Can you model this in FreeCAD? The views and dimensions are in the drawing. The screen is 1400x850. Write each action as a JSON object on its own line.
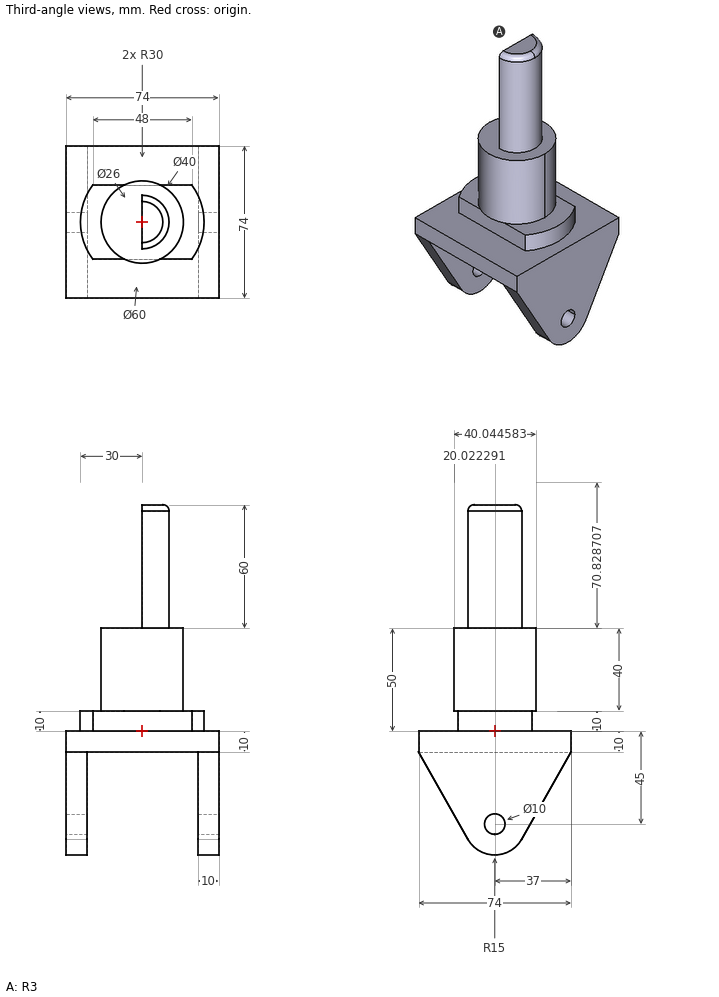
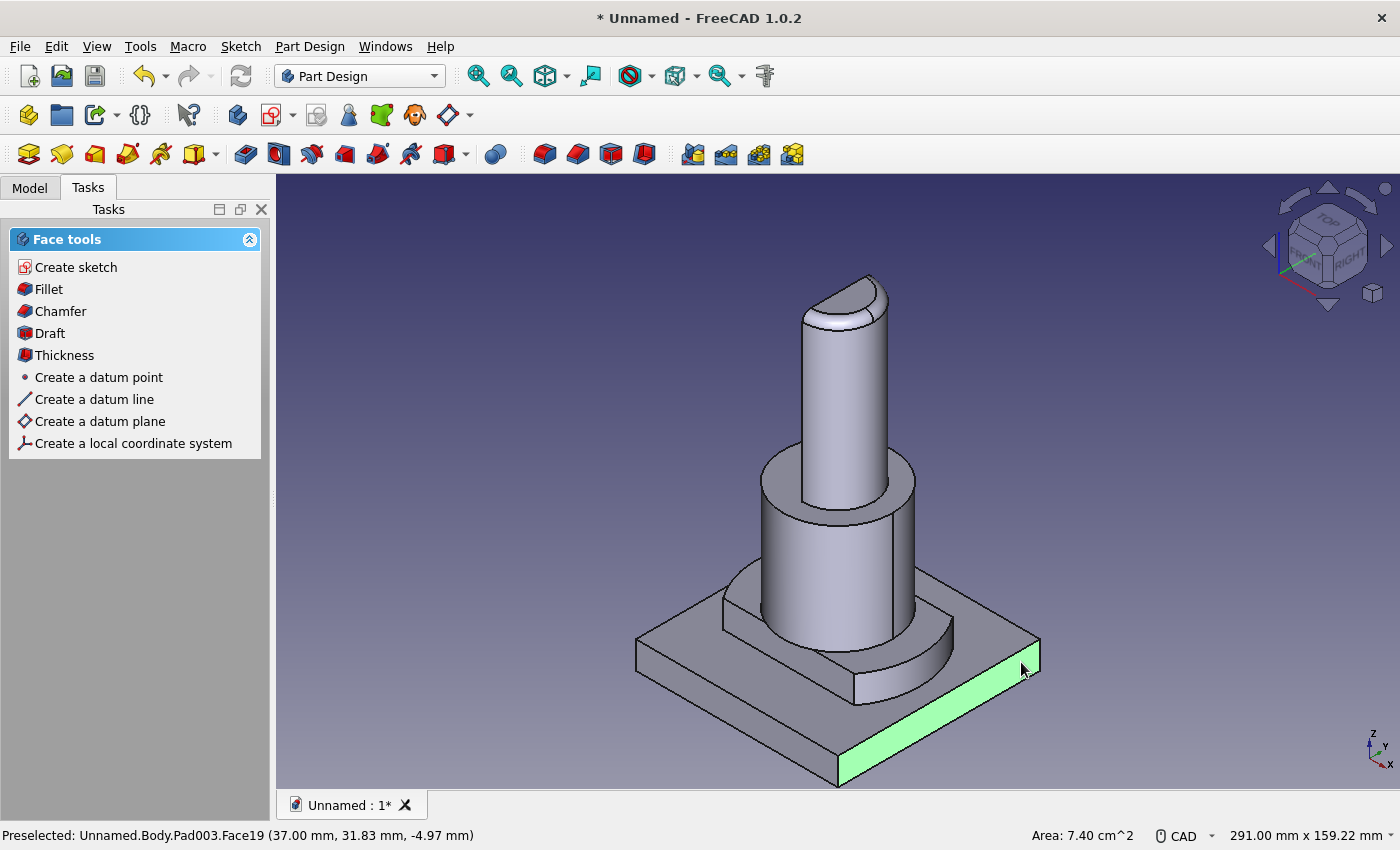
{"action": "left_click", "coordinate": [270, 116]}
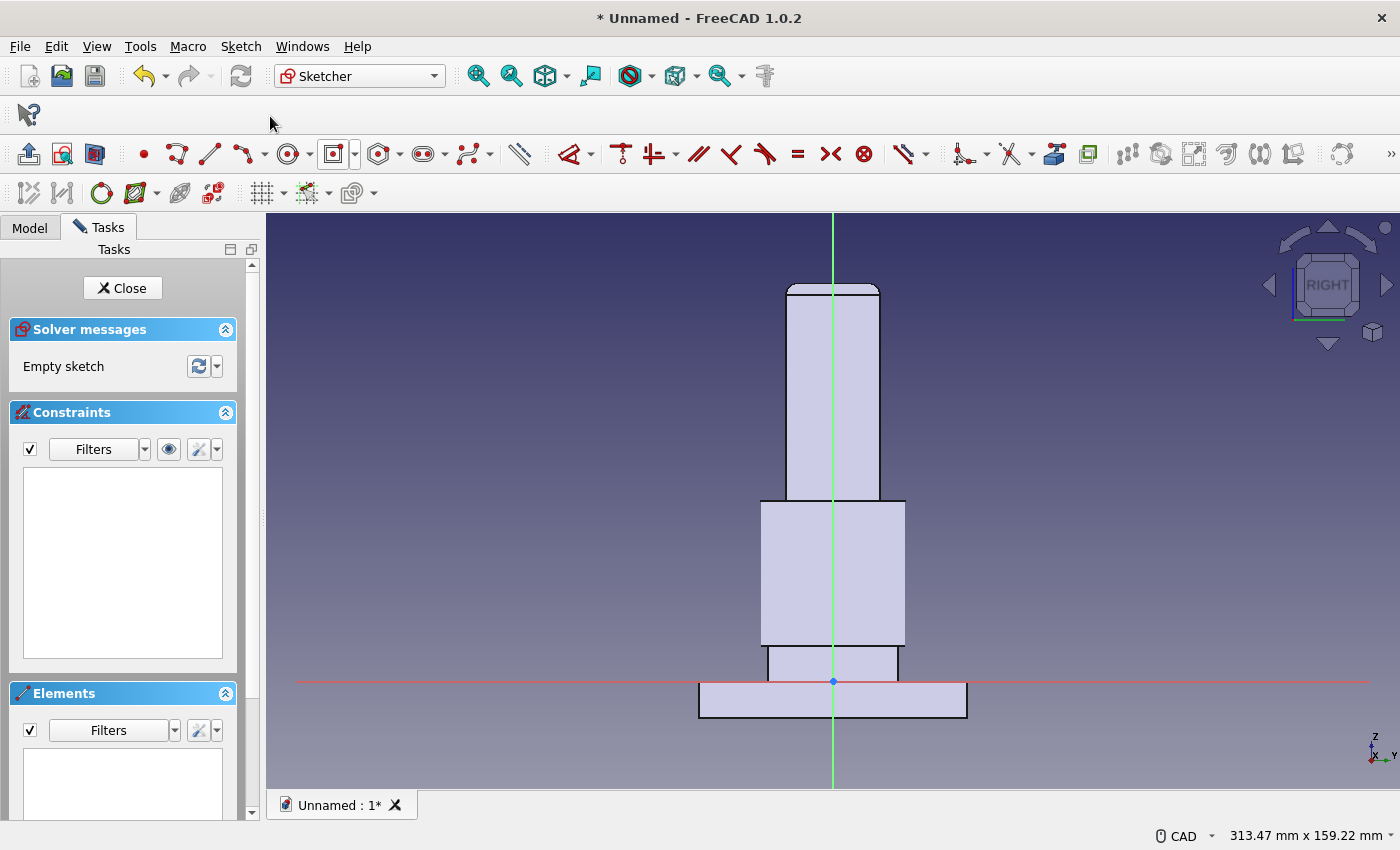
{"action": "scroll", "coordinate": [764, 501], "scroll_direction": "down", "scroll_amount": 5}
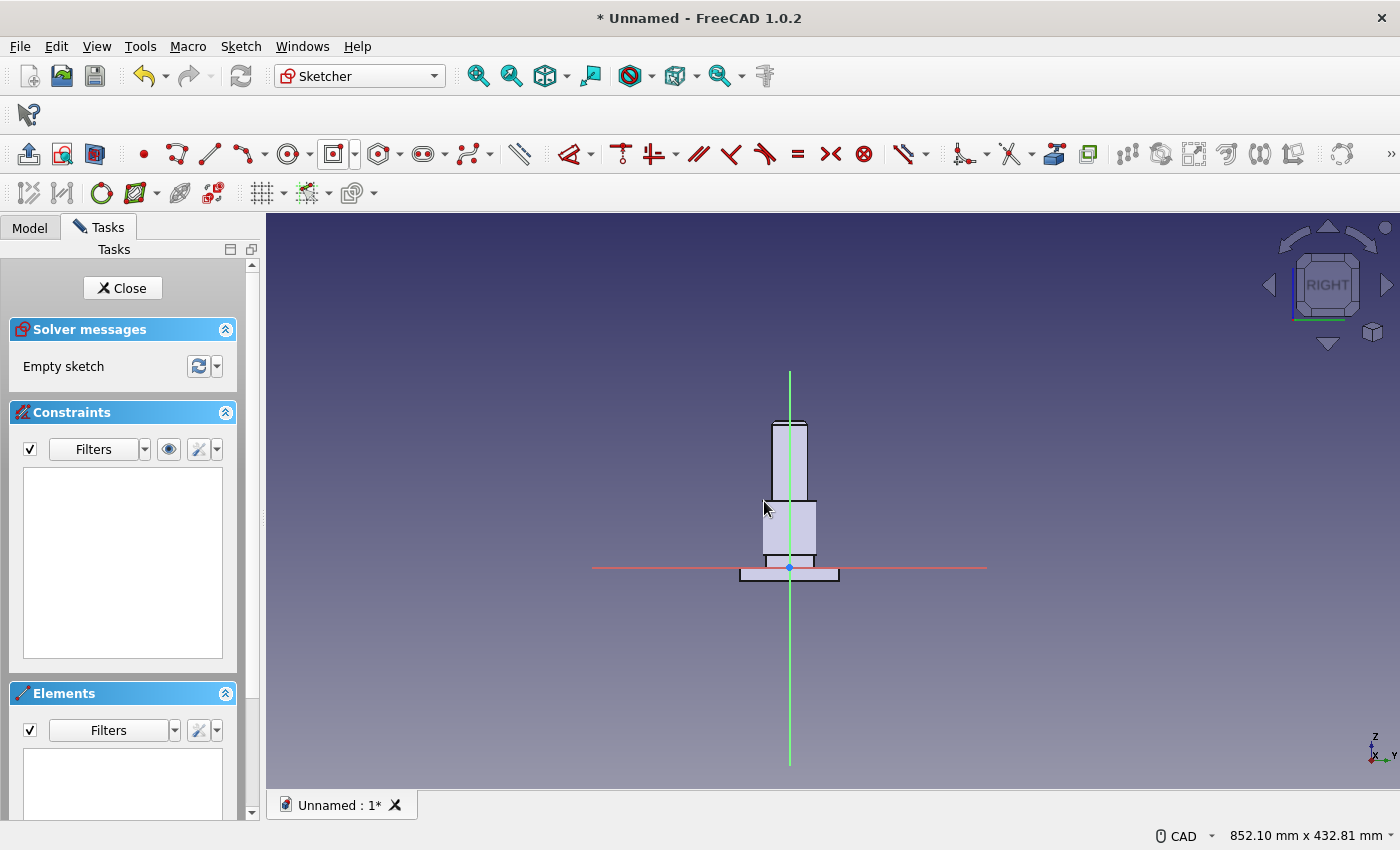
{"action": "scroll", "coordinate": [796, 635], "scroll_direction": "up", "scroll_amount": 8}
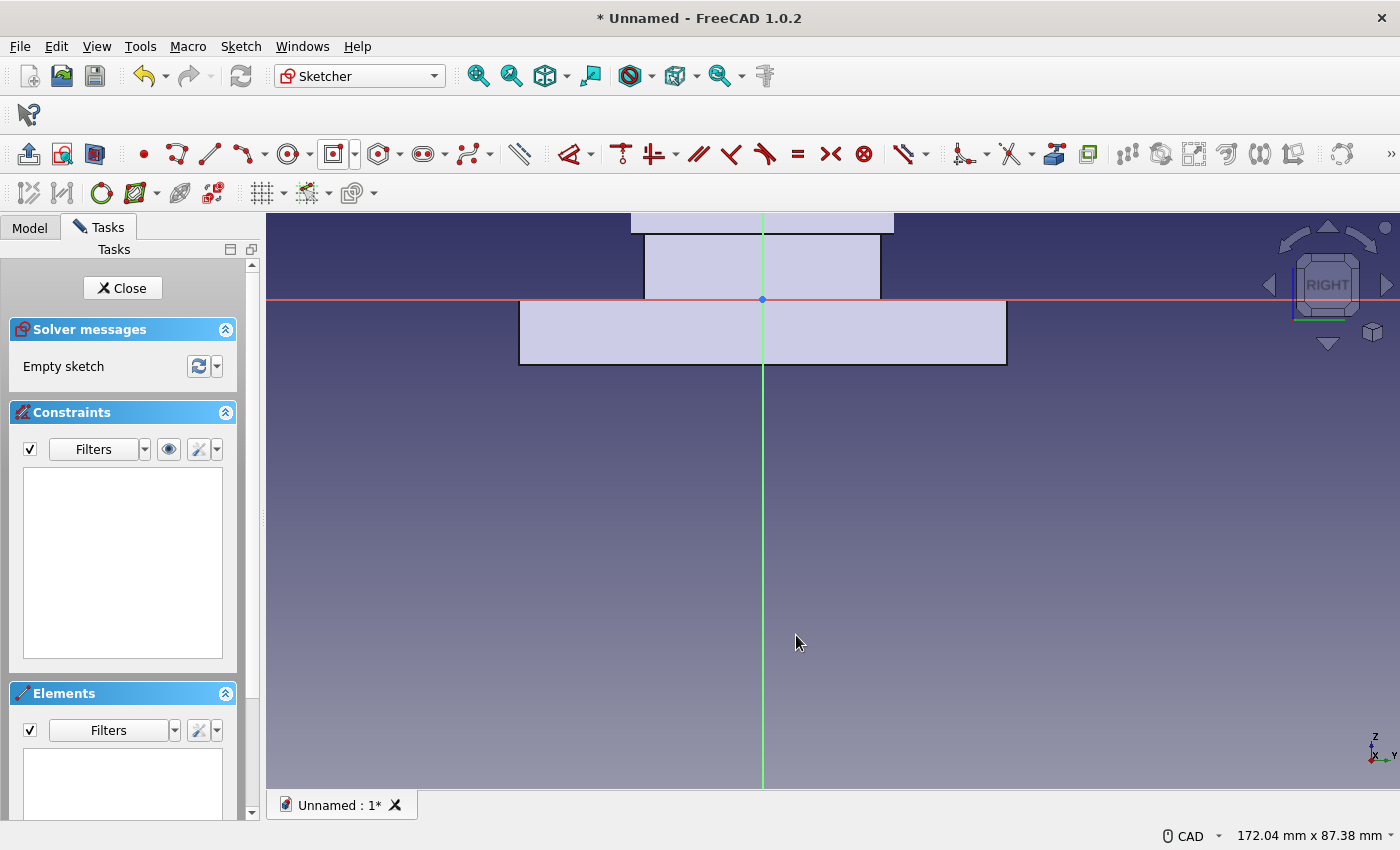
{"action": "key", "text": "g m"}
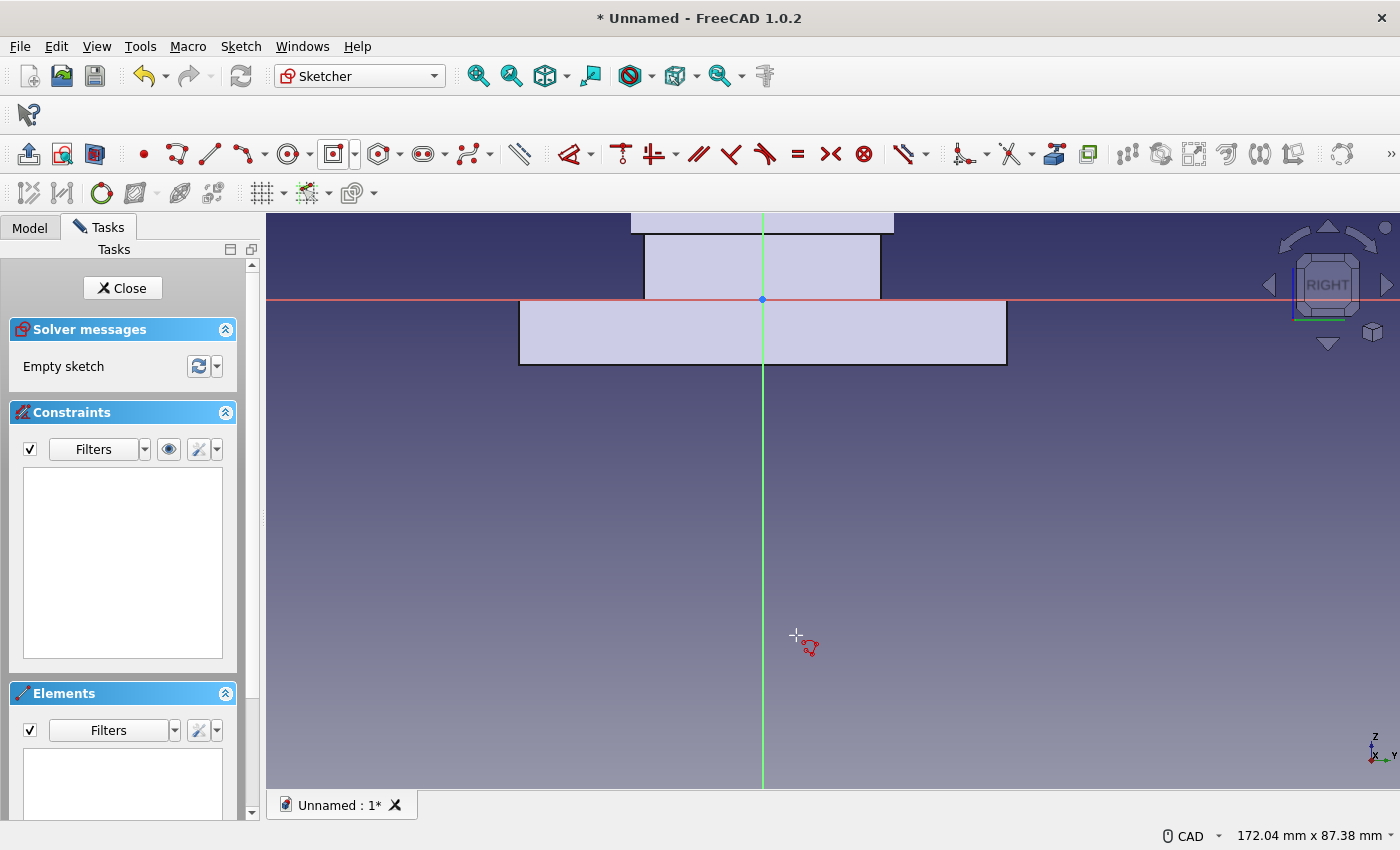
{"action": "left_click", "coordinate": [849, 645]}
{"action": "left_click", "coordinate": [1007, 365]}
{"action": "left_click", "coordinate": [519, 365]}
{"action": "left_click", "coordinate": [677, 645]}
{"action": "right_click", "coordinate": [677, 645]}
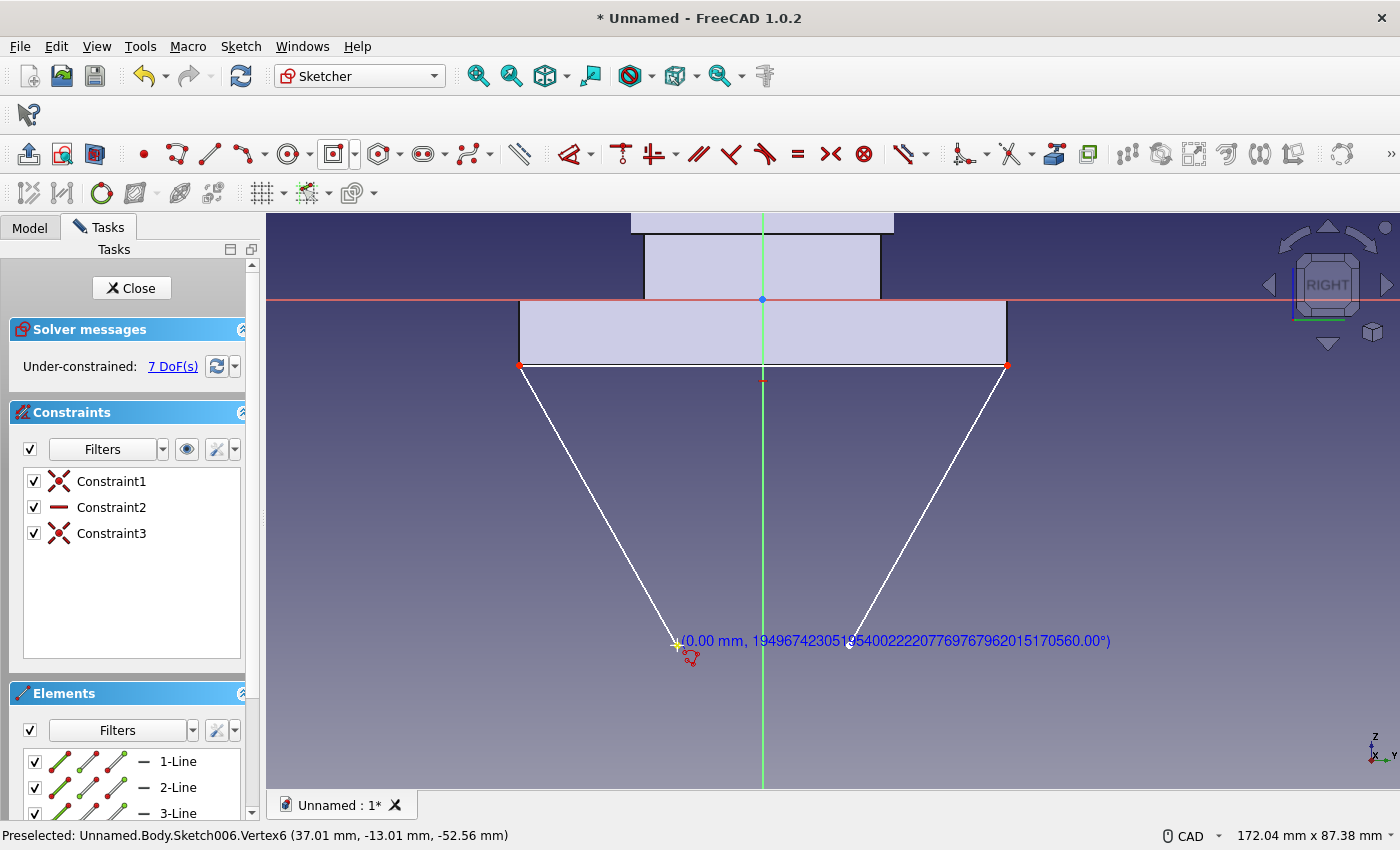
{"action": "key", "text": "g 3 a"}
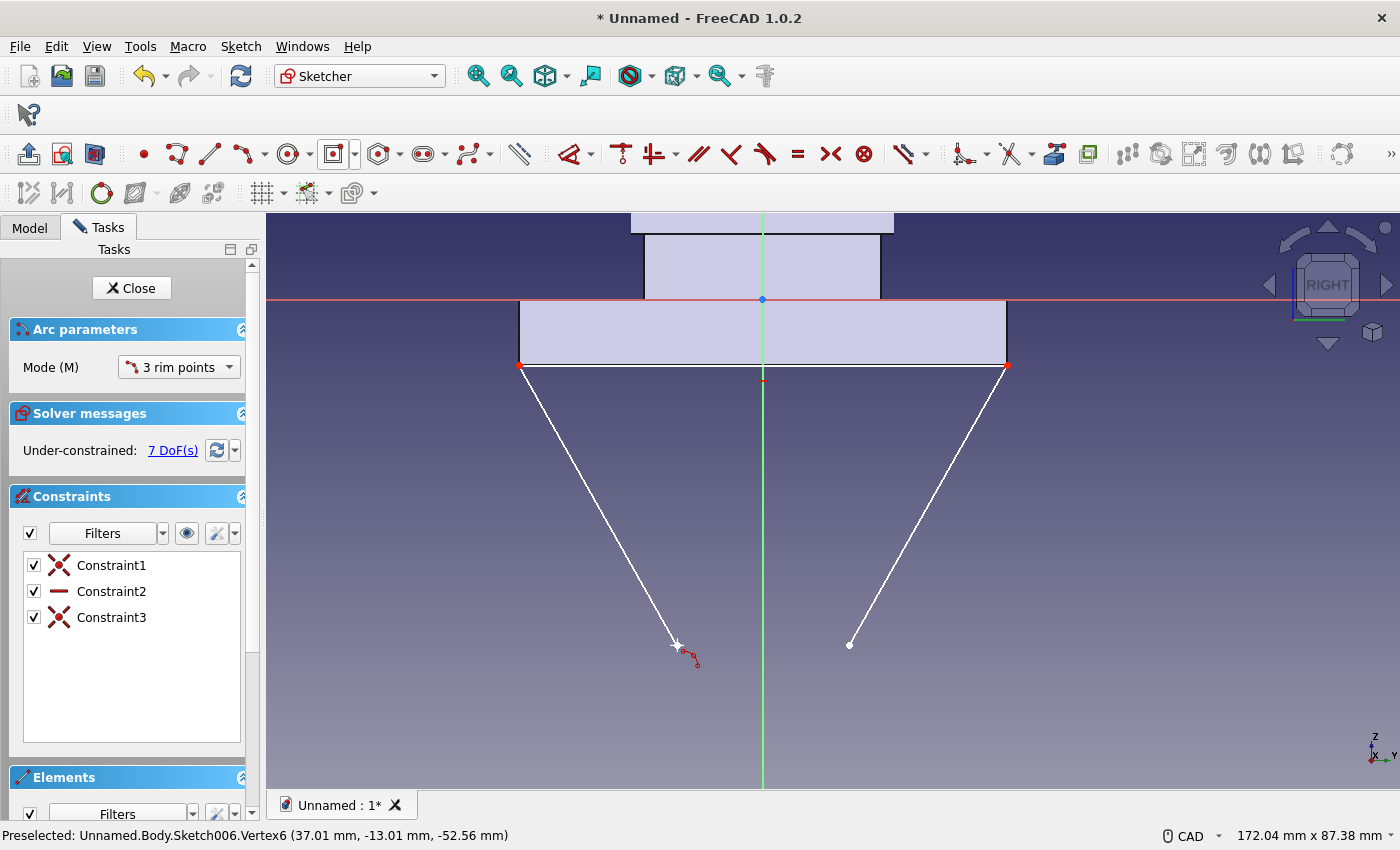
{"action": "left_click", "coordinate": [677, 646]}
{"action": "left_click", "coordinate": [849, 646]}
{"action": "left_click", "coordinate": [742, 693]}
{"action": "key", "text": "Escape"}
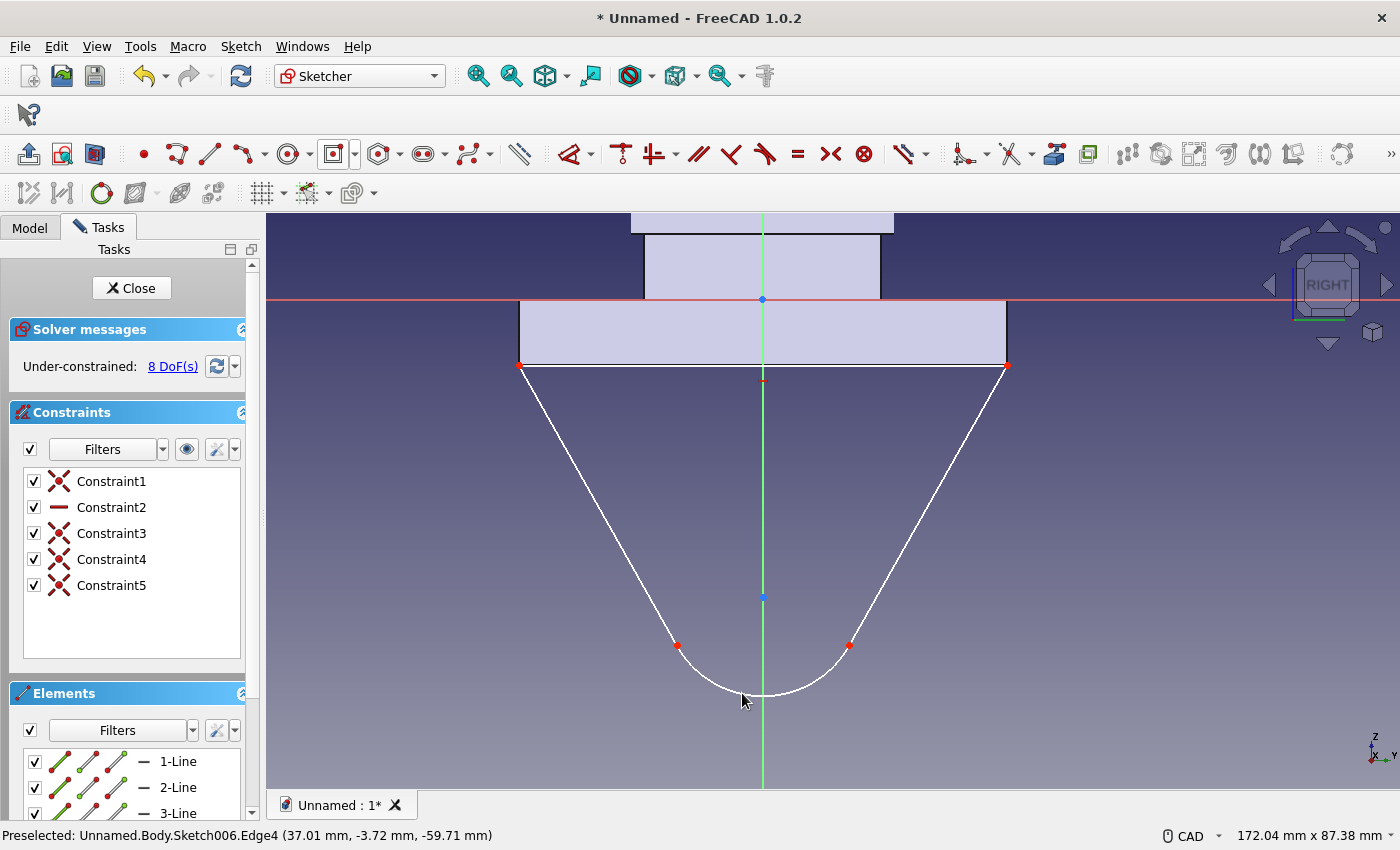
{"action": "left_click", "coordinate": [896, 562]}